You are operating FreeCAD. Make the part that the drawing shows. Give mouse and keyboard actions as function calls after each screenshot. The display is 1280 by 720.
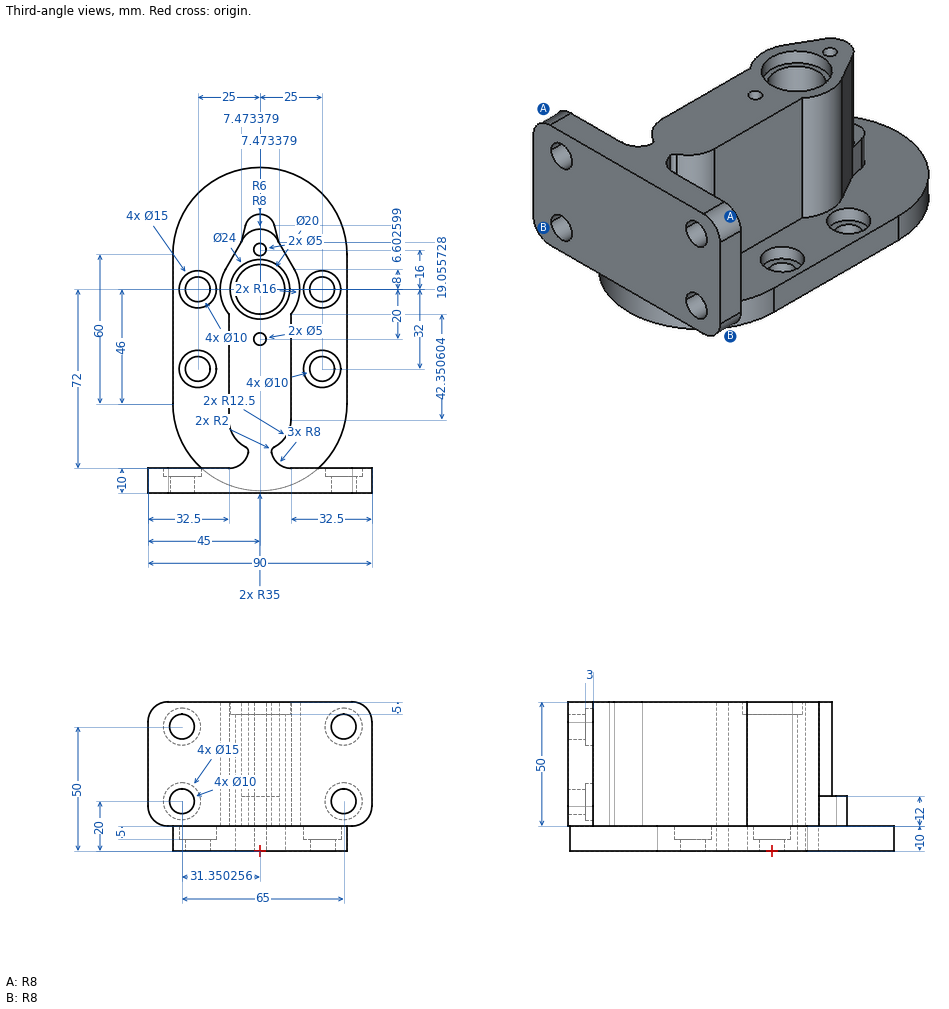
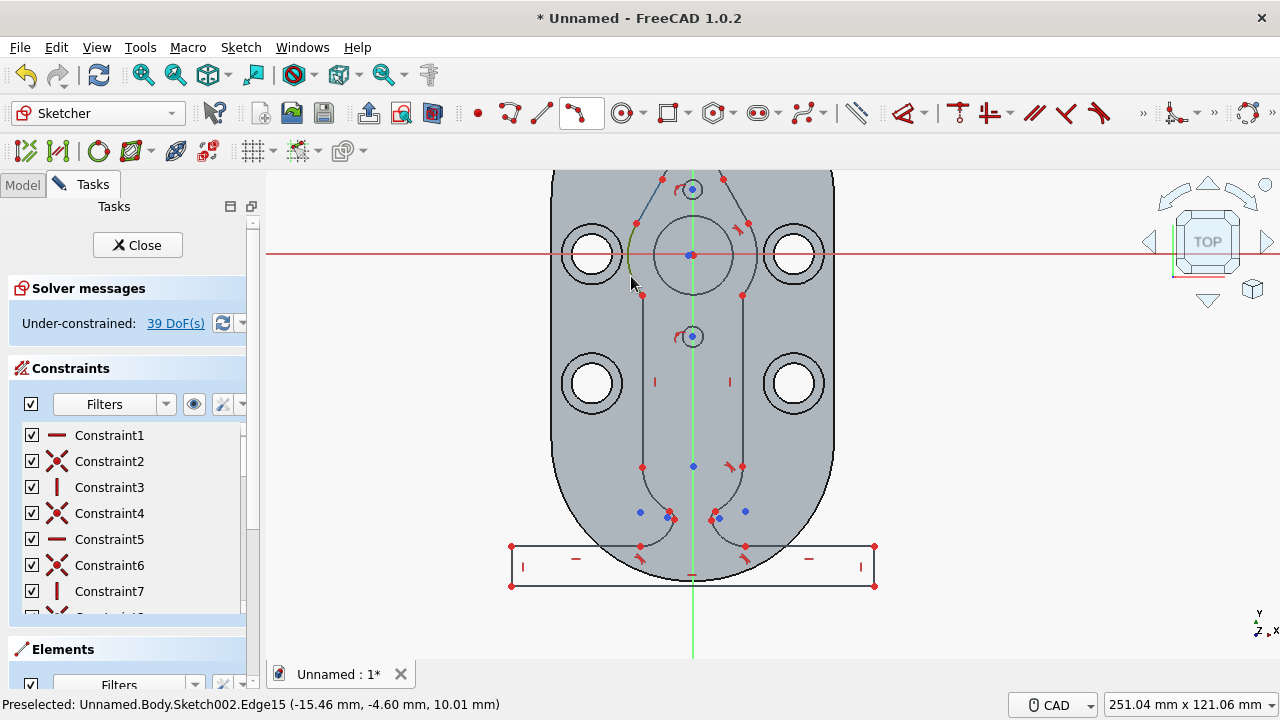
click(1100, 114)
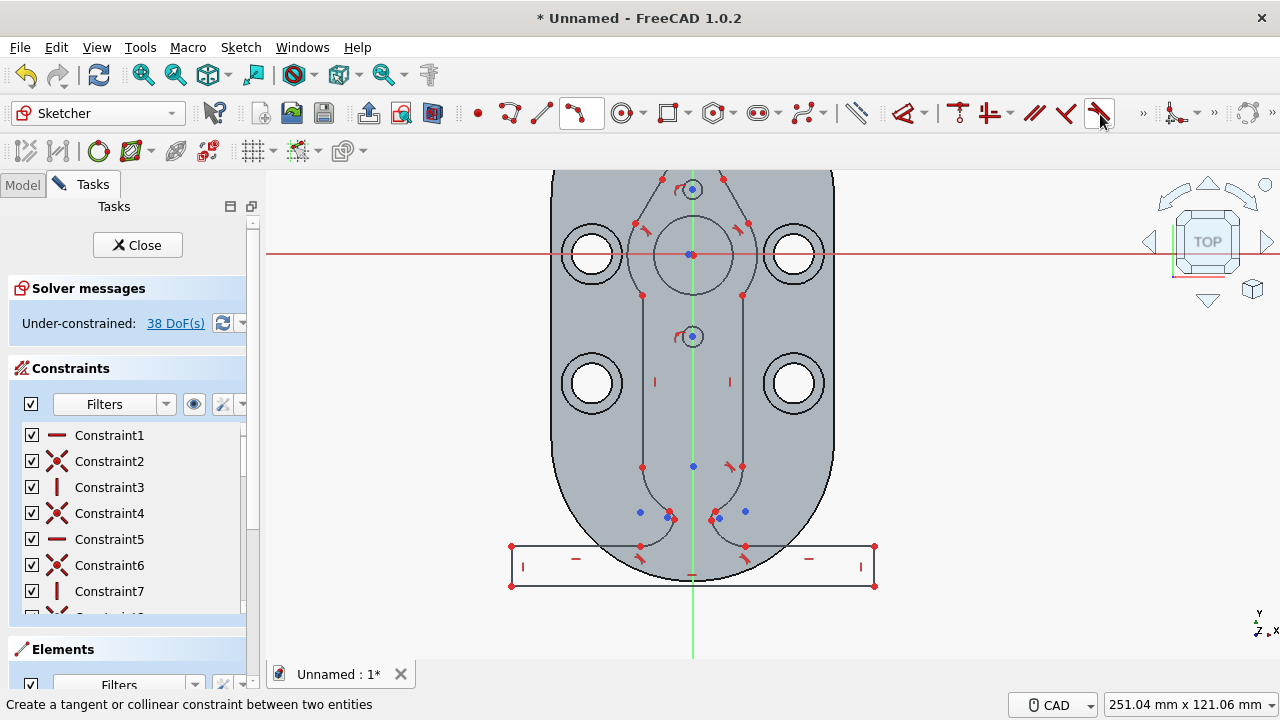
click(643, 347)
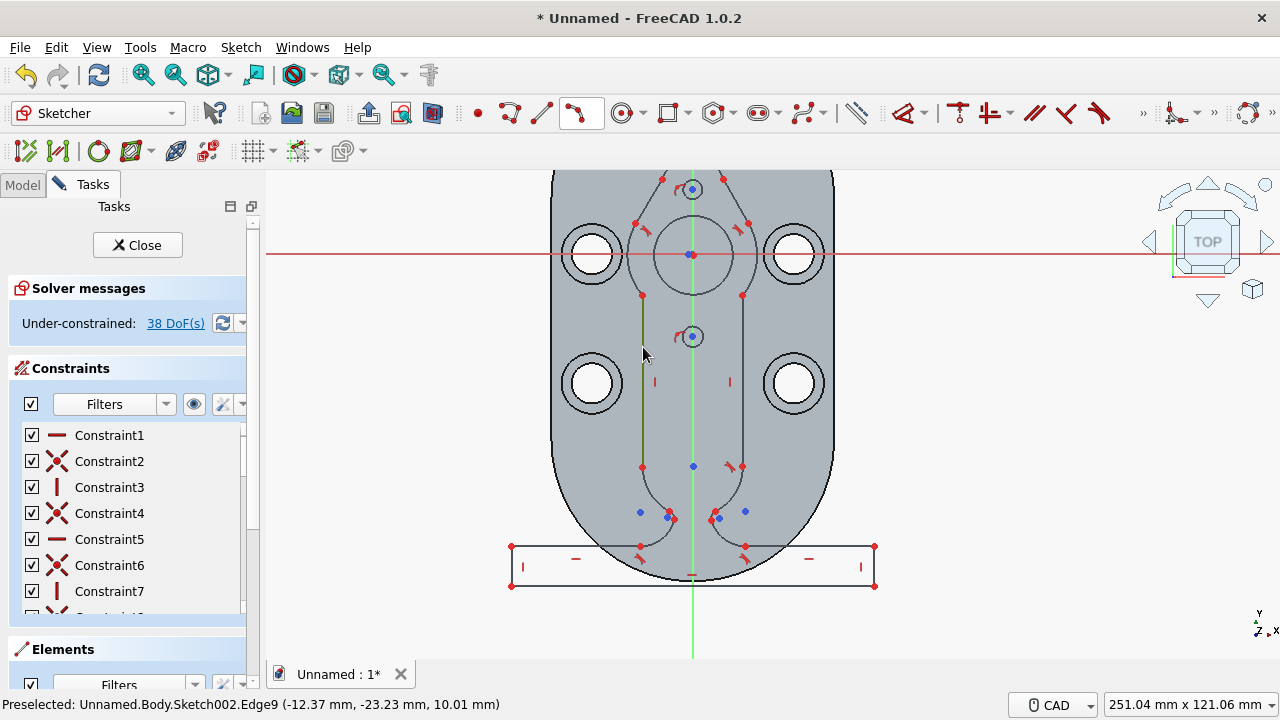
click(646, 483)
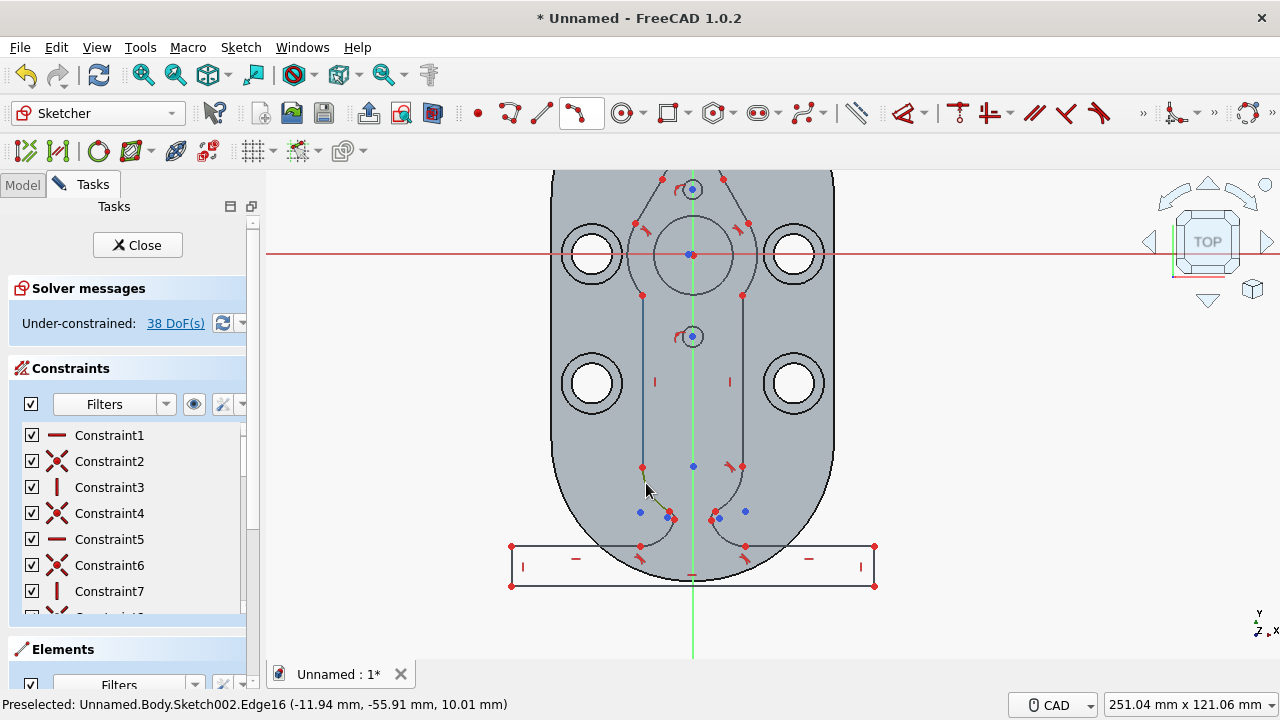
click(1100, 114)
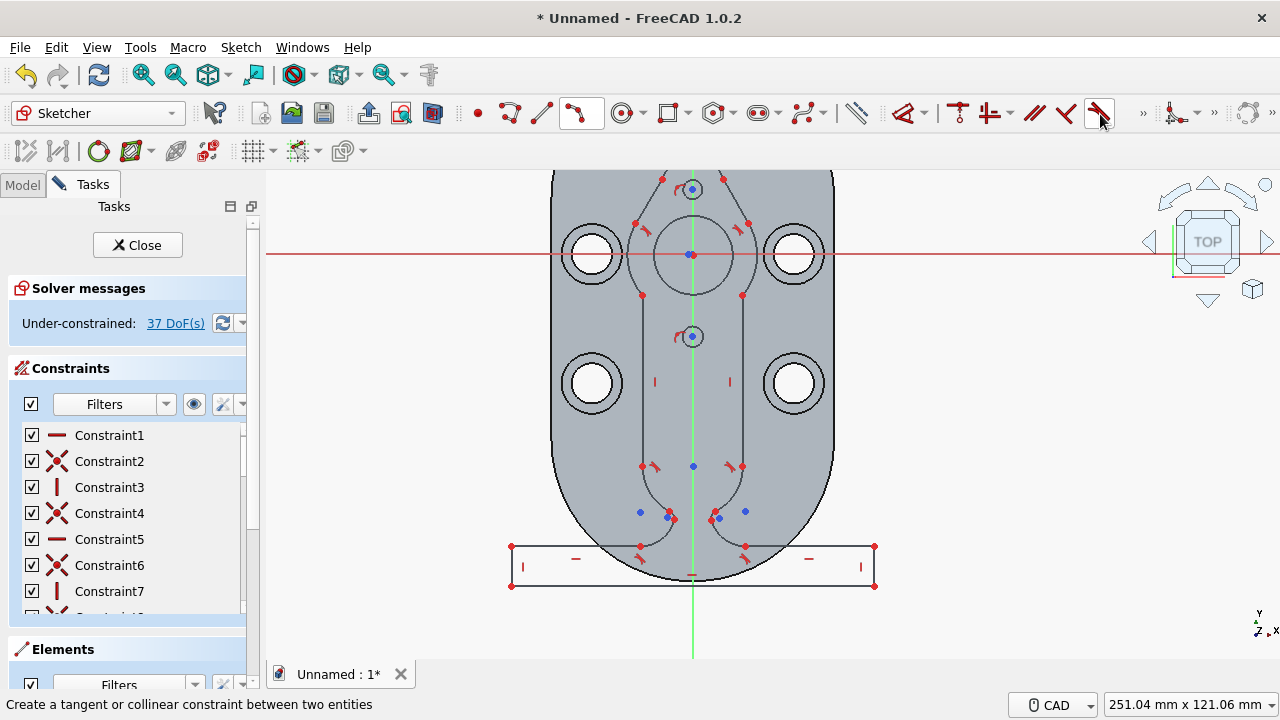
click(718, 533)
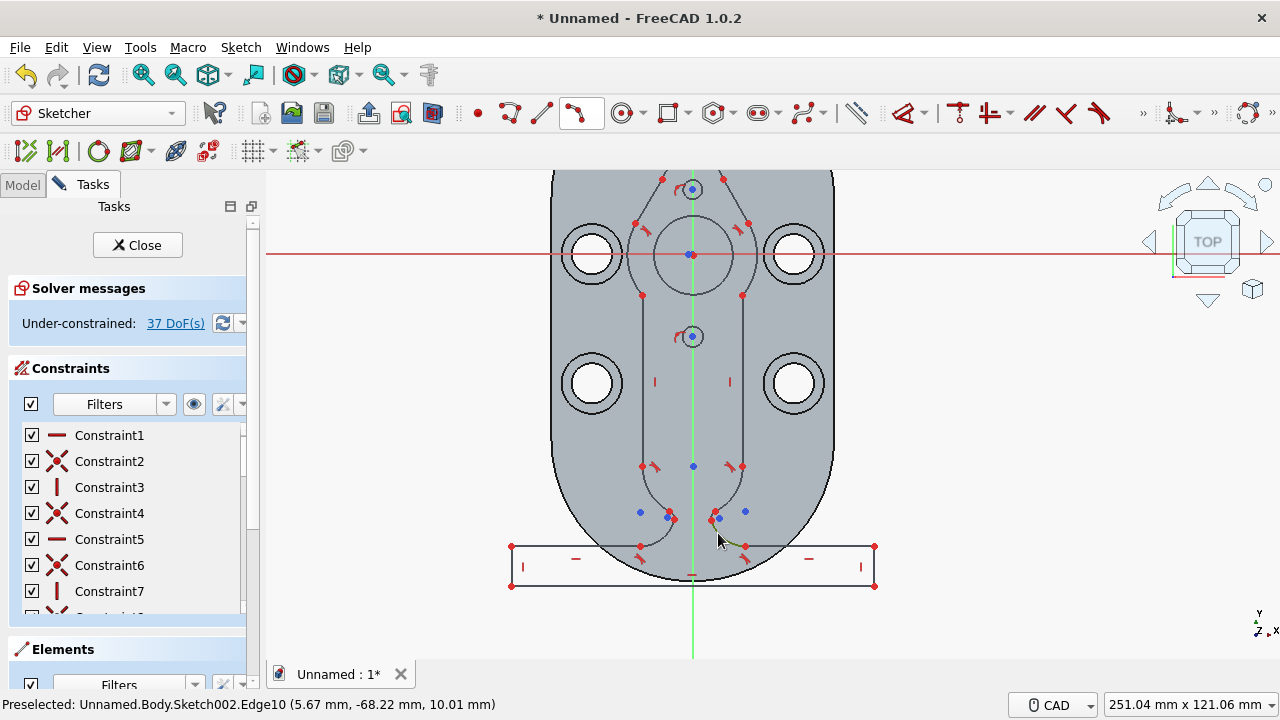
scroll(712, 515, up, 5)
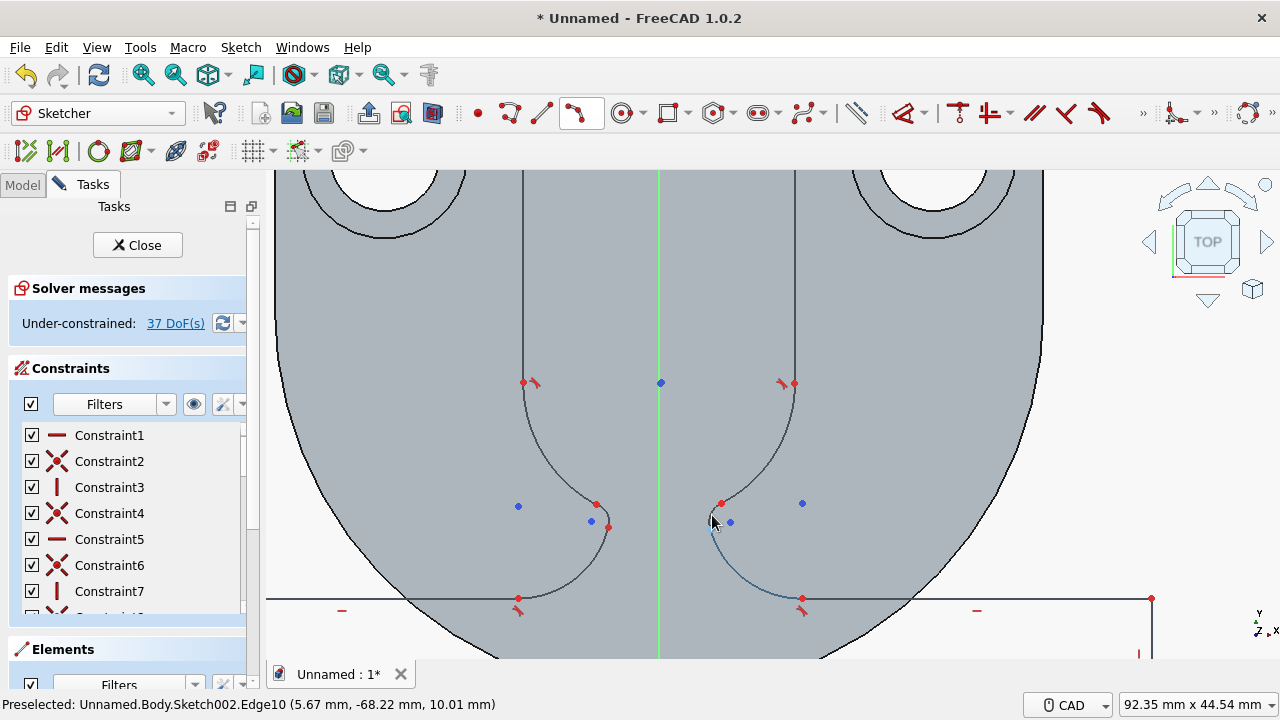
click(711, 514)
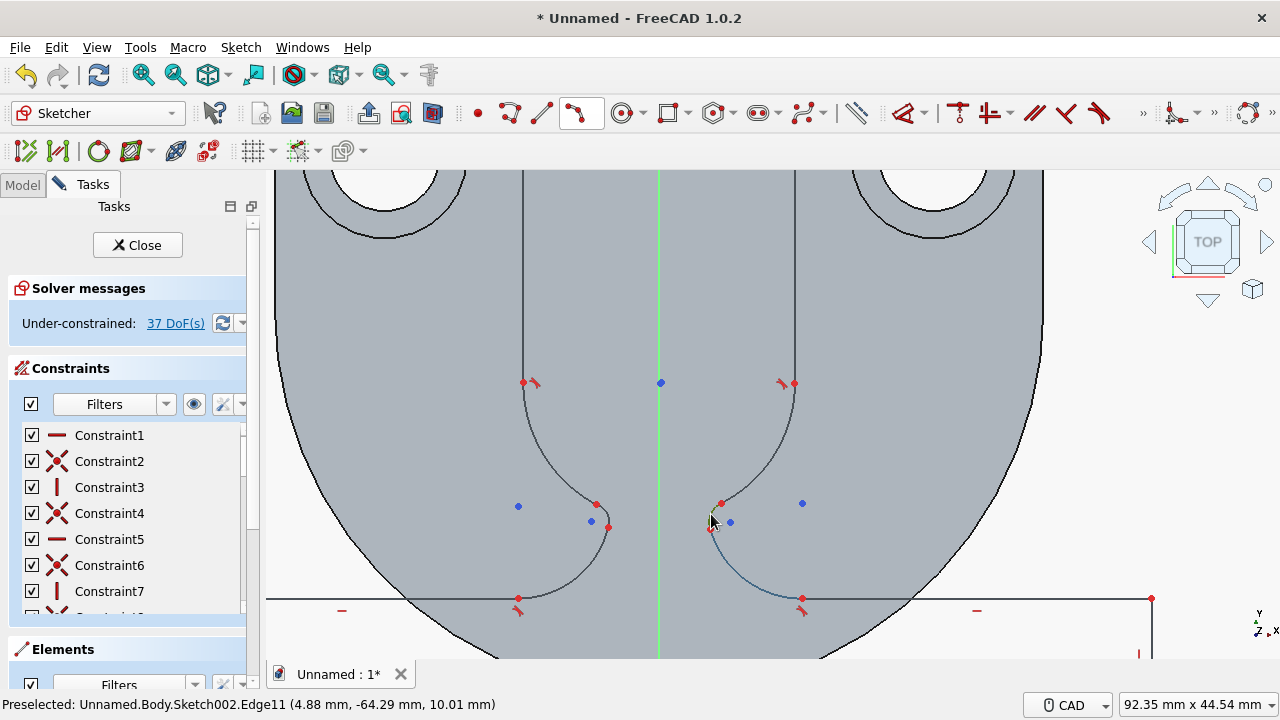
click(1100, 114)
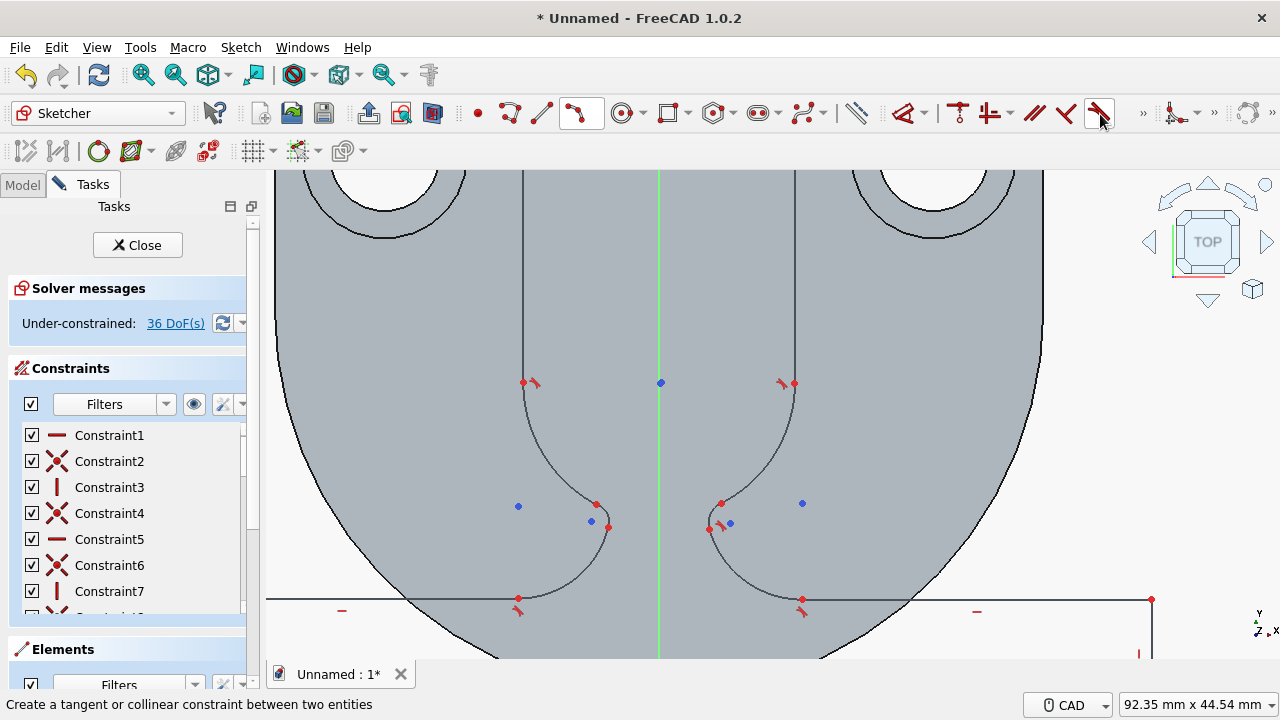
scroll(714, 509, up, 2)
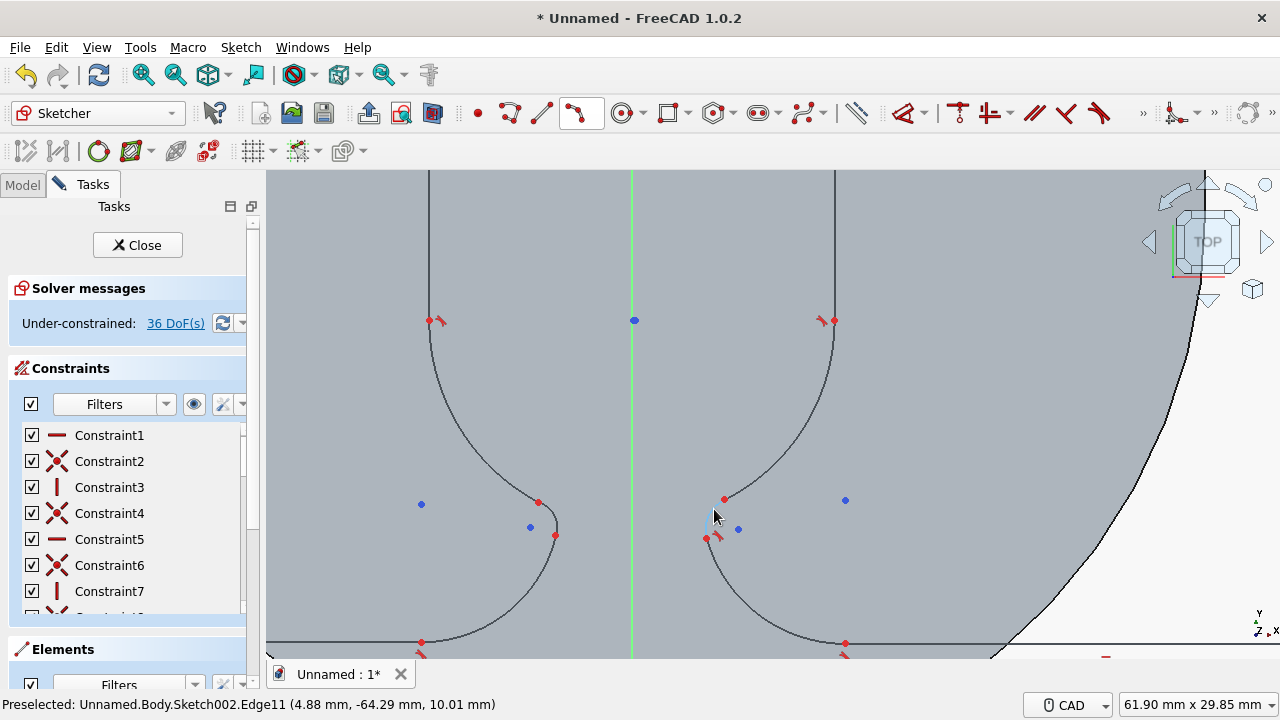
click(714, 508)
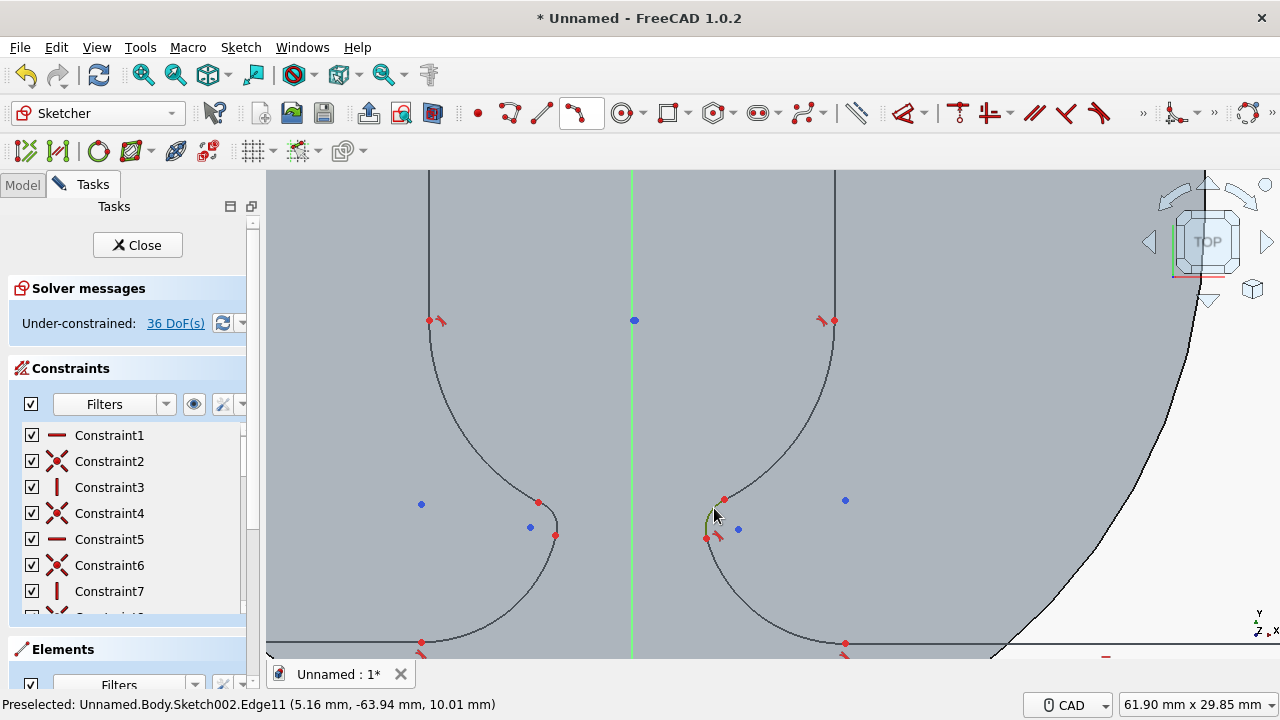
scroll(719, 510, down, 9)